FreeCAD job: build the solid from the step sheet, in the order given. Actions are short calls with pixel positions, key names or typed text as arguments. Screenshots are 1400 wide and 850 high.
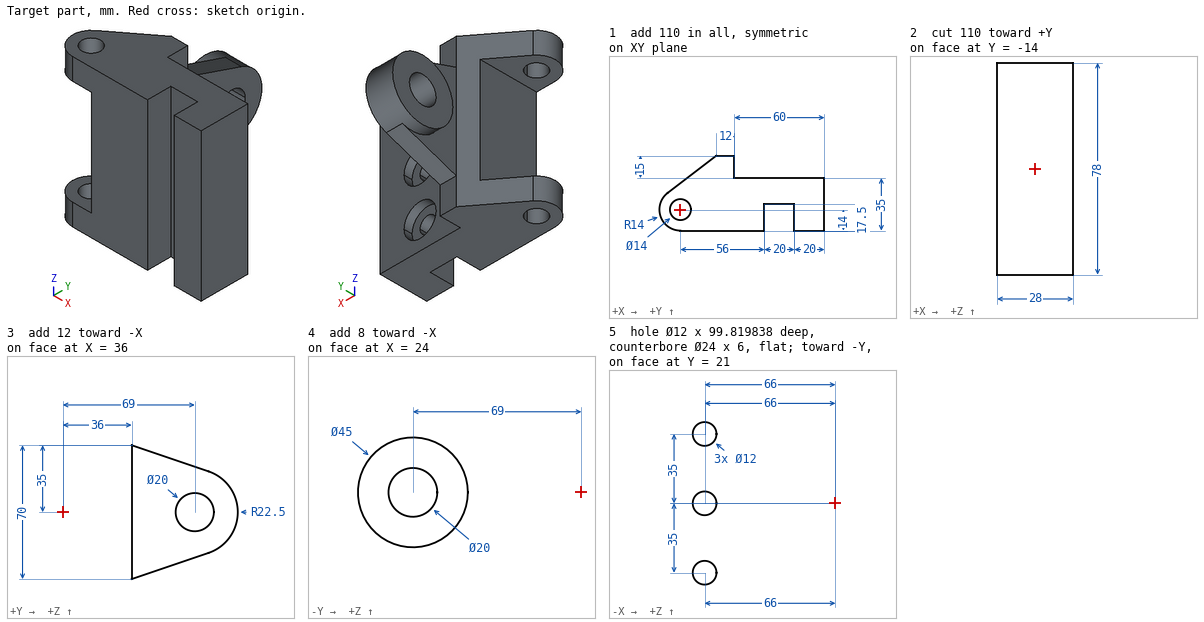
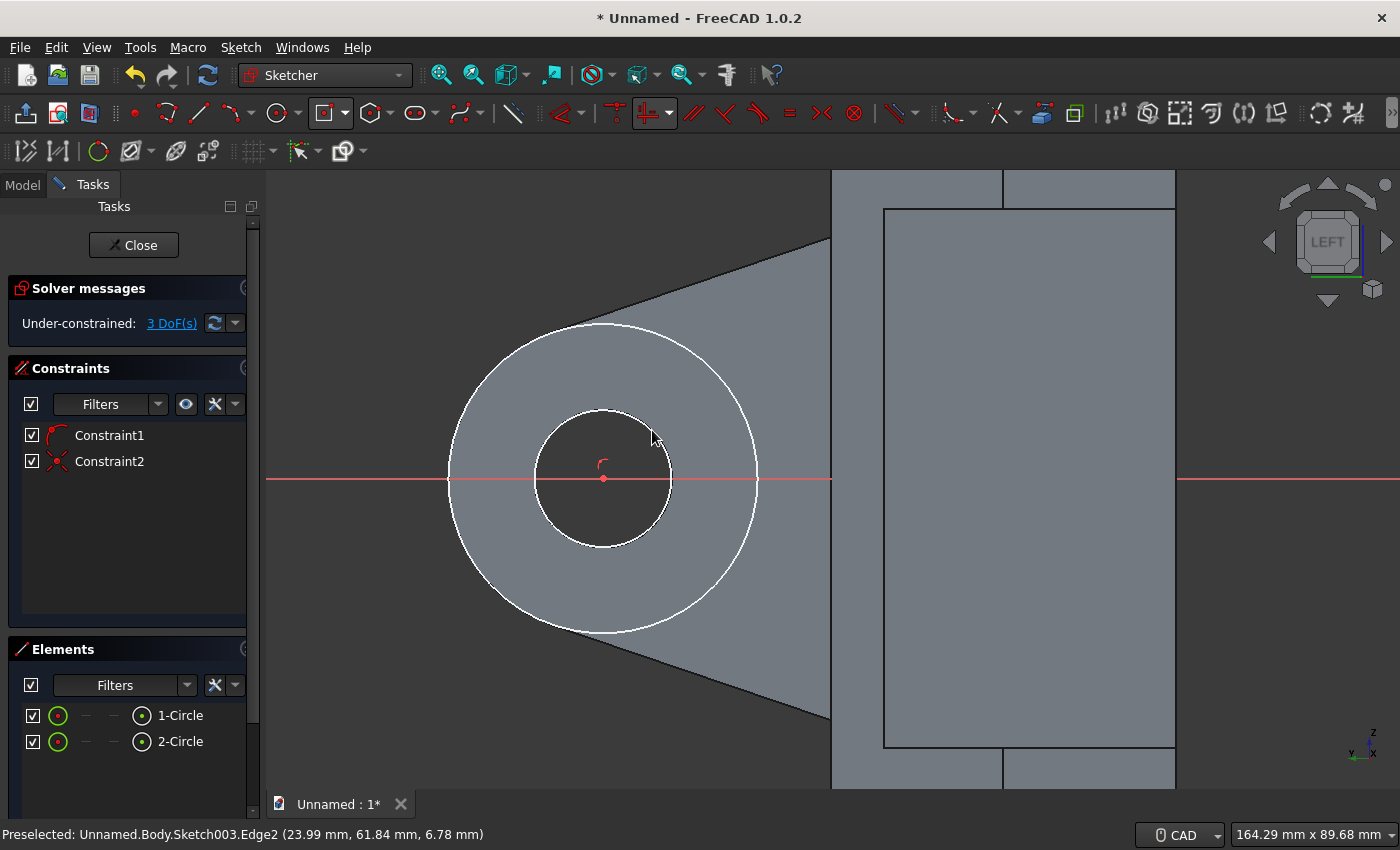
click(560, 114)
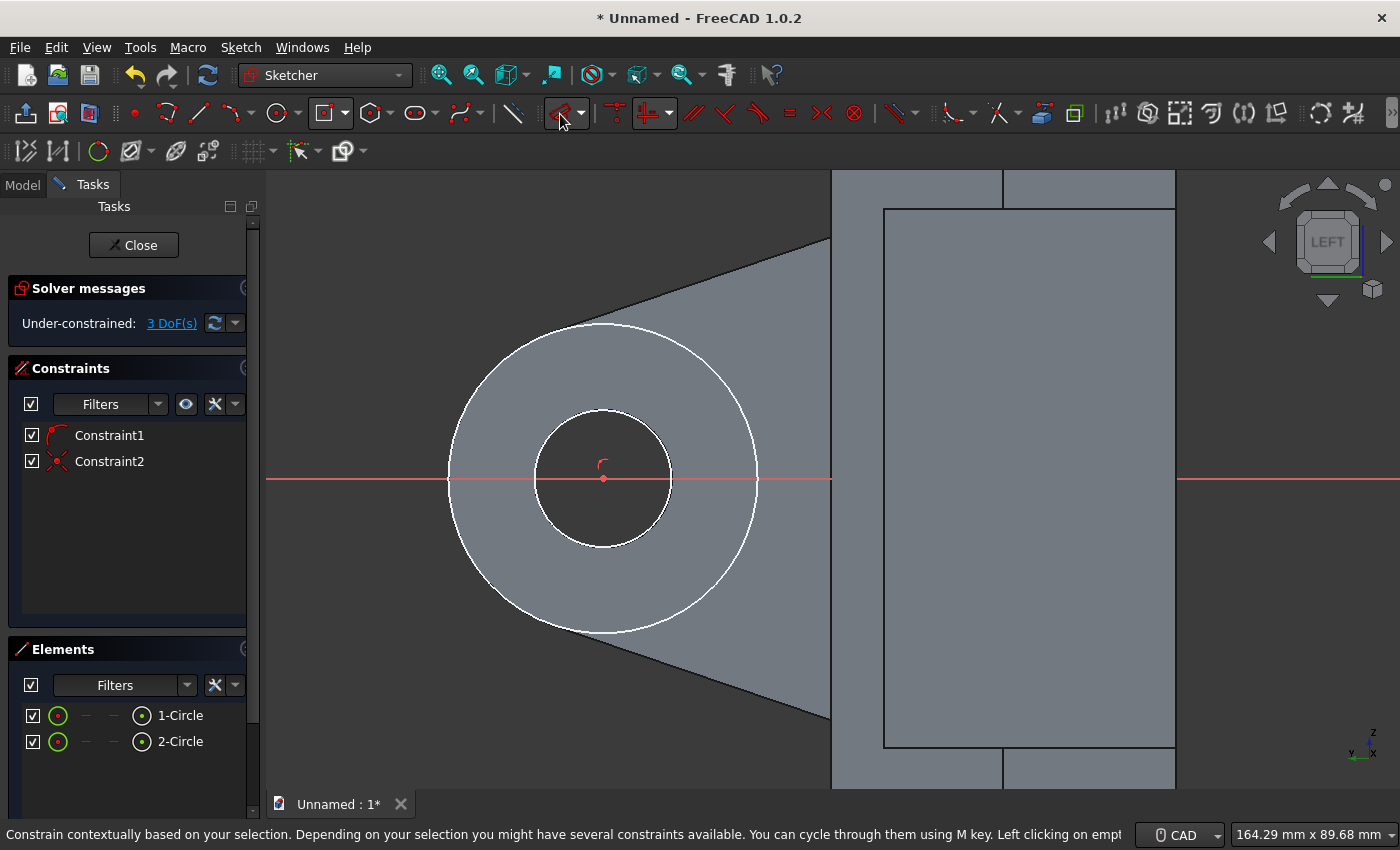
click(712, 369)
click(735, 346)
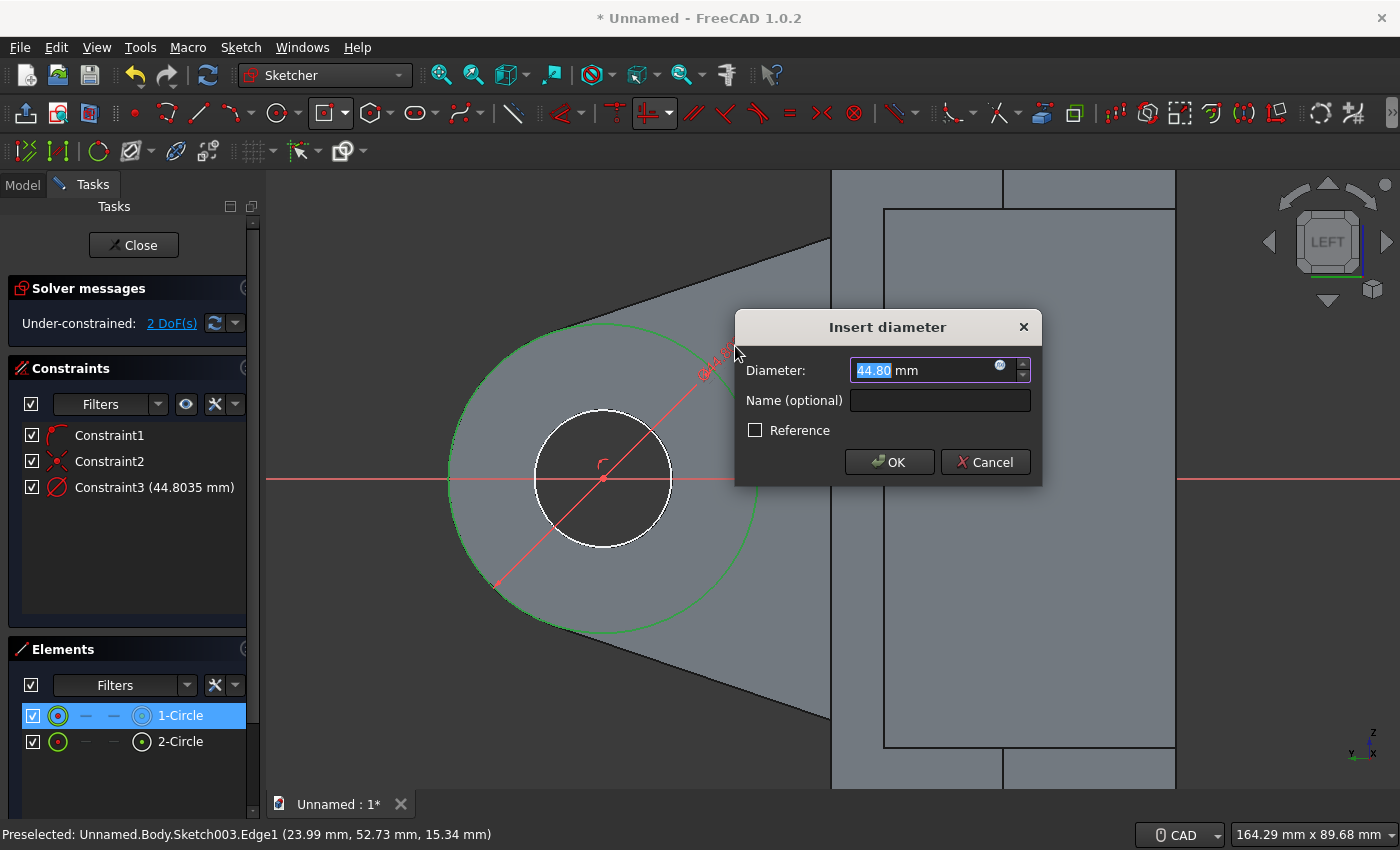
text(45)
key(Return)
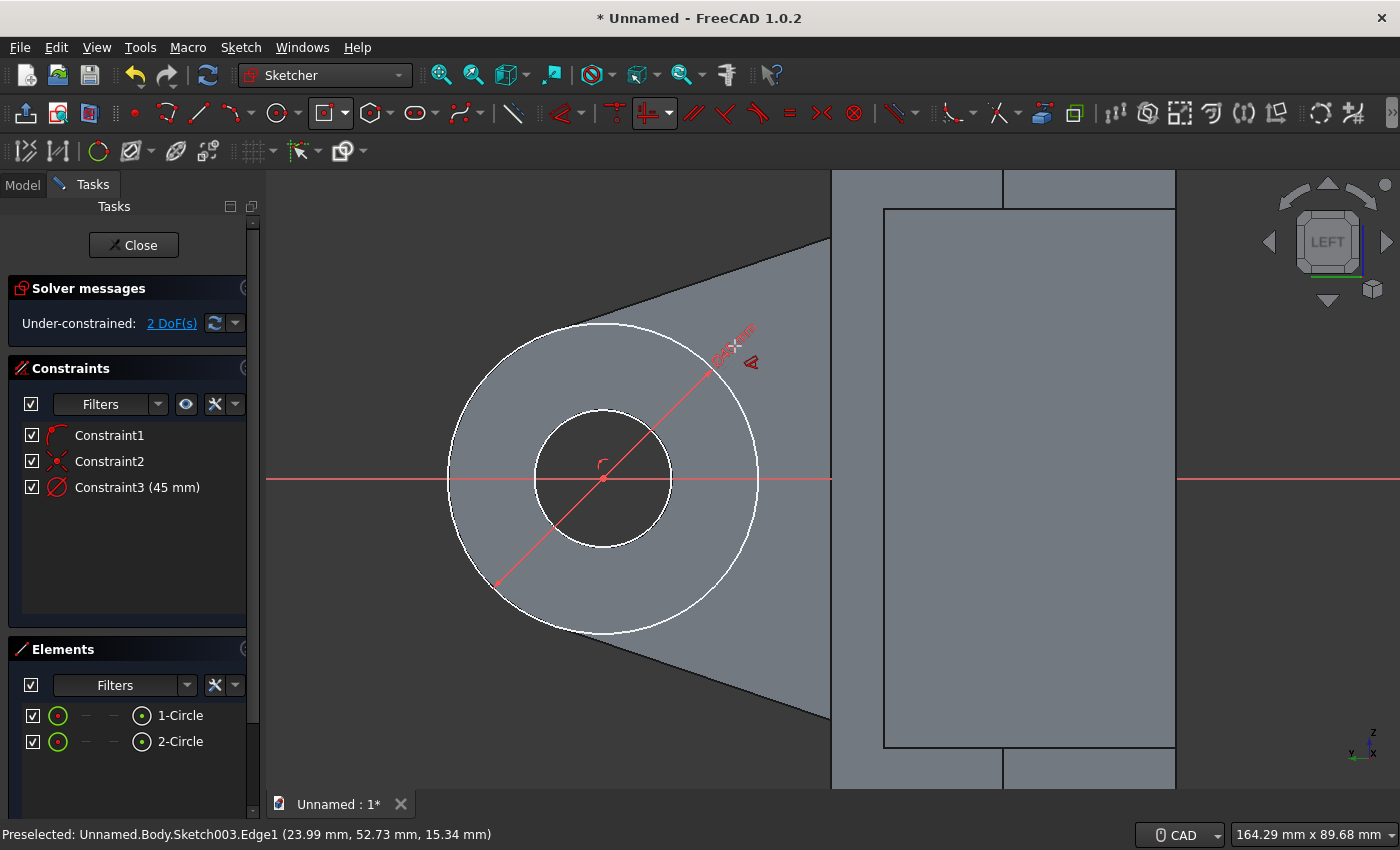
click(651, 430)
click(673, 407)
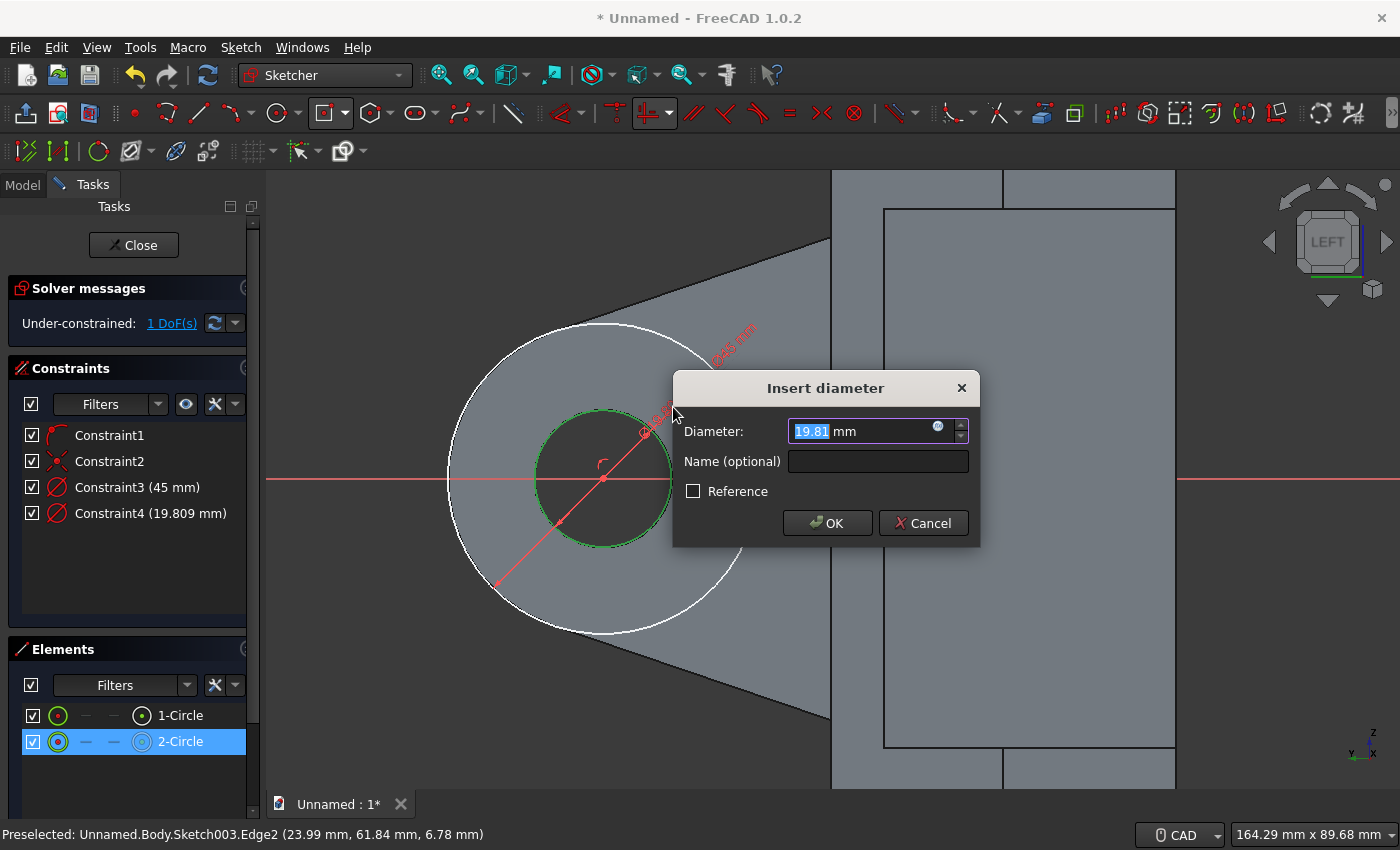
text(20)
key(Return)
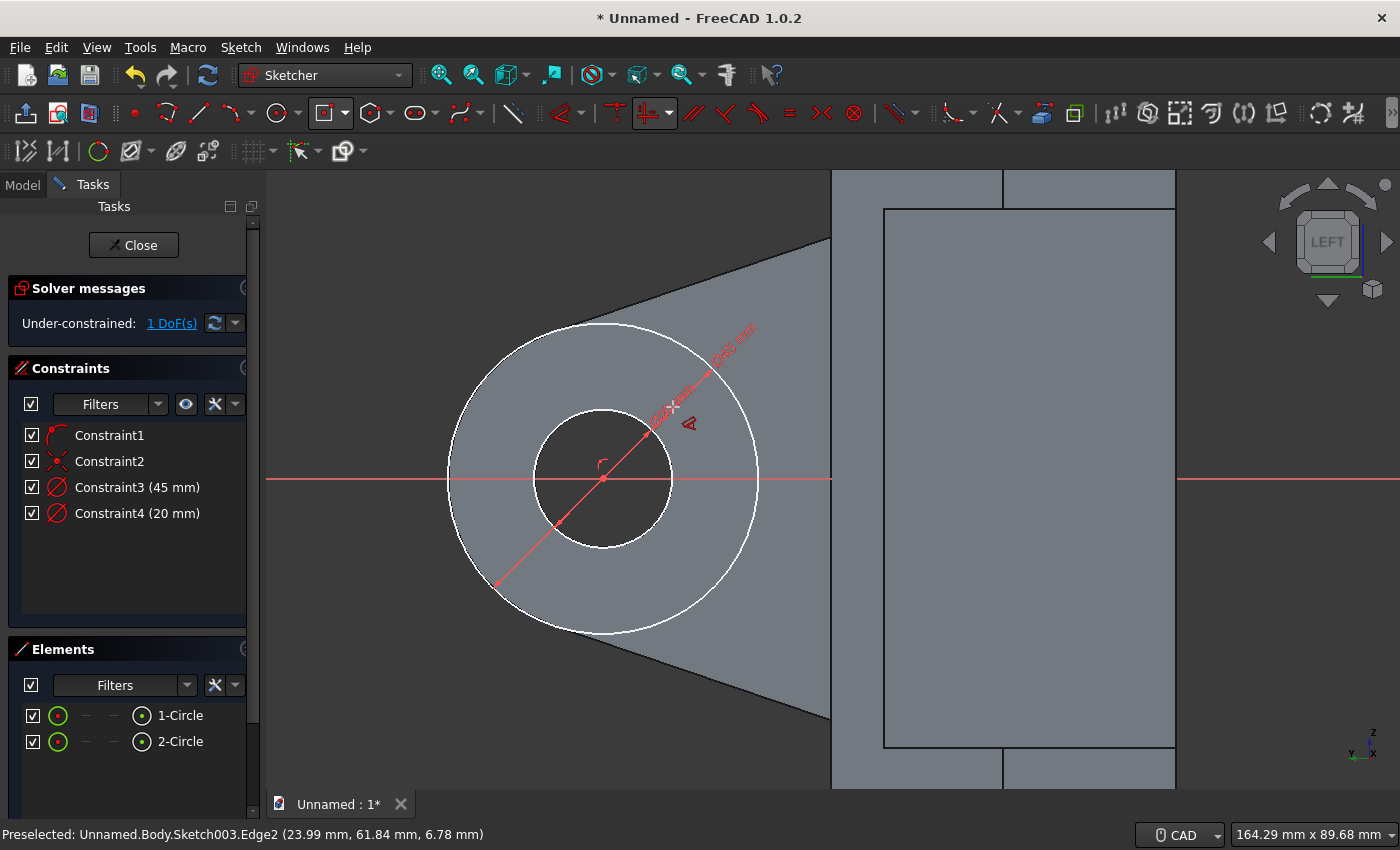
click(603, 479)
click(841, 513)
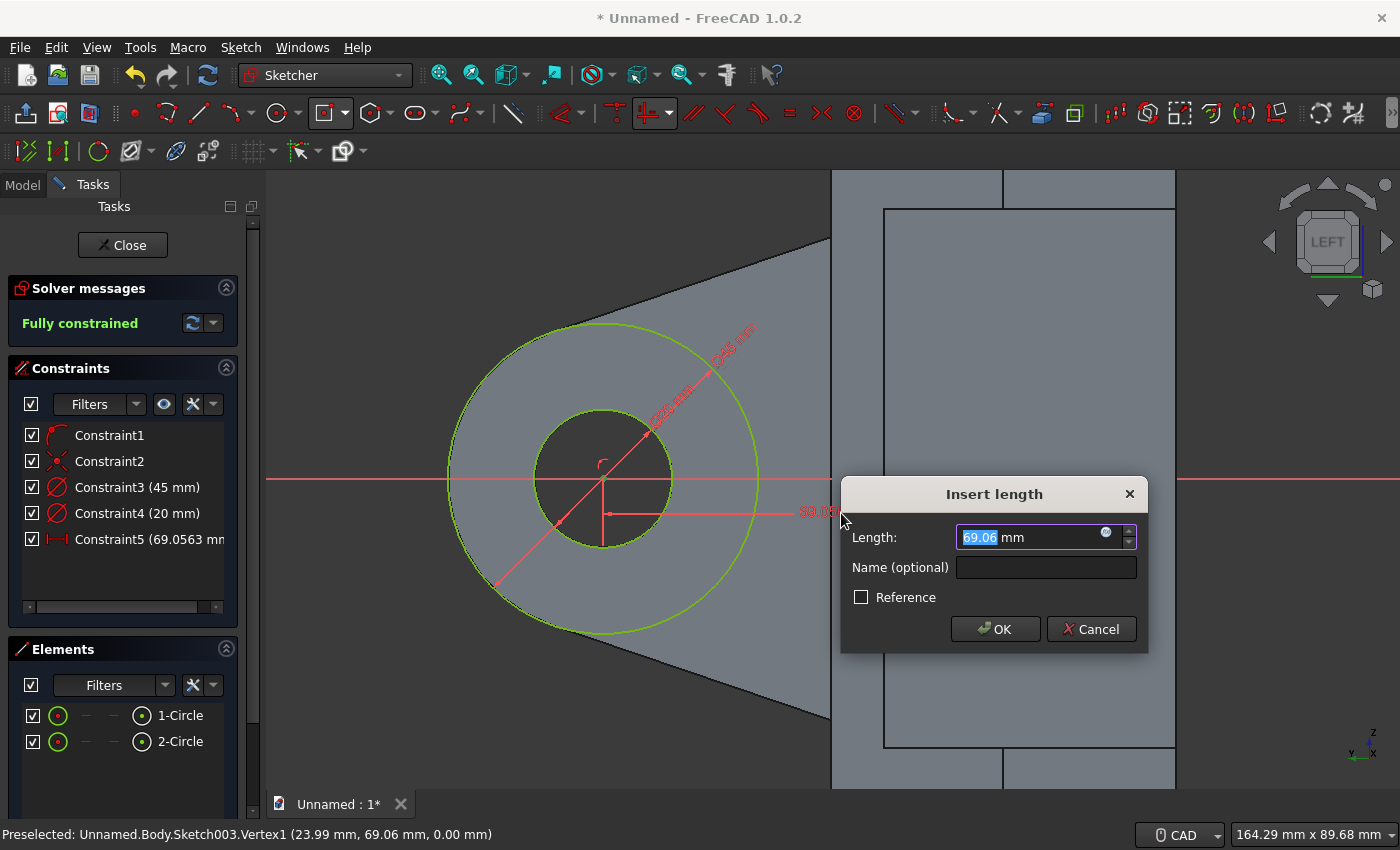
text(69)
key(Return)
key(Escape)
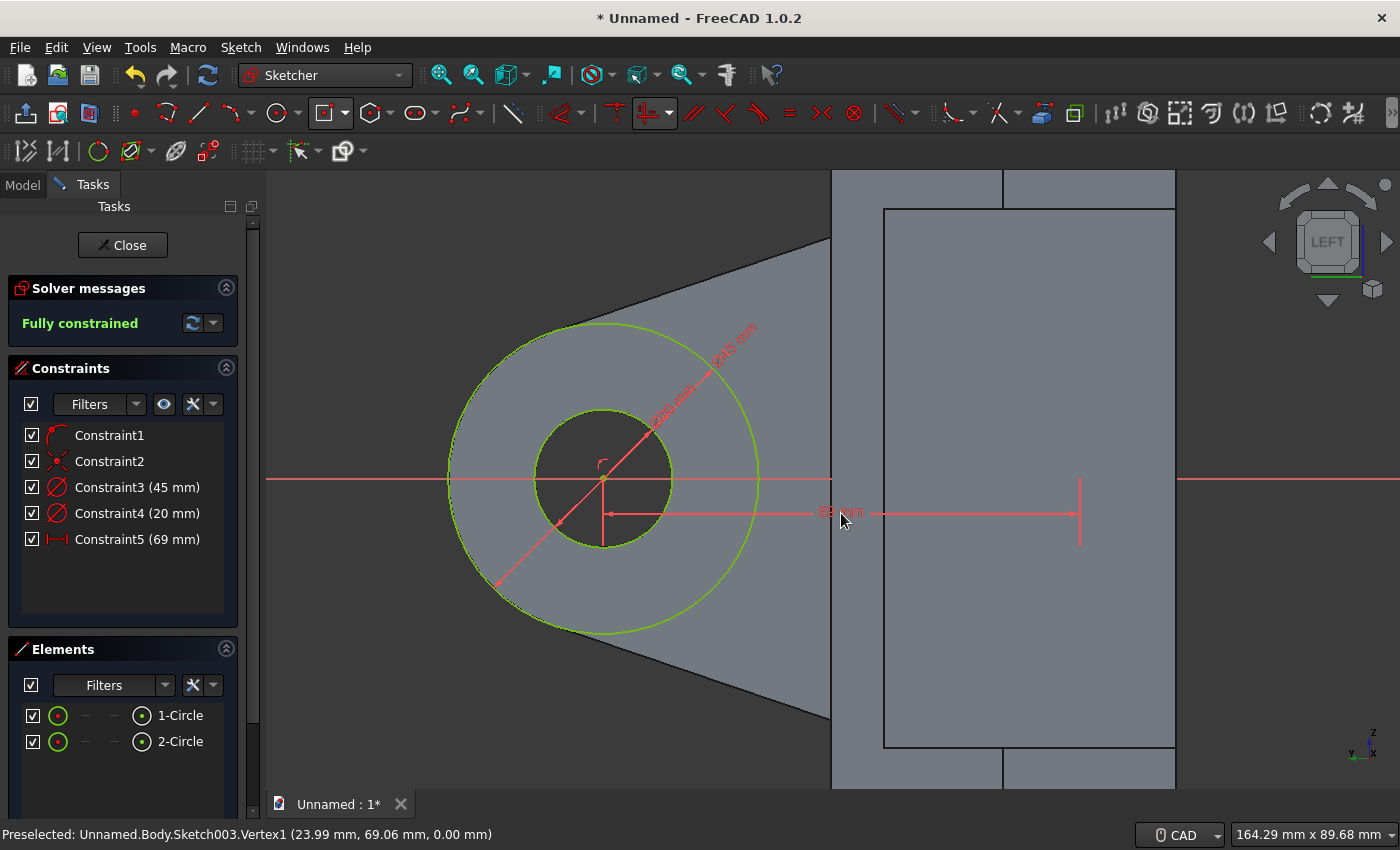
click(123, 245)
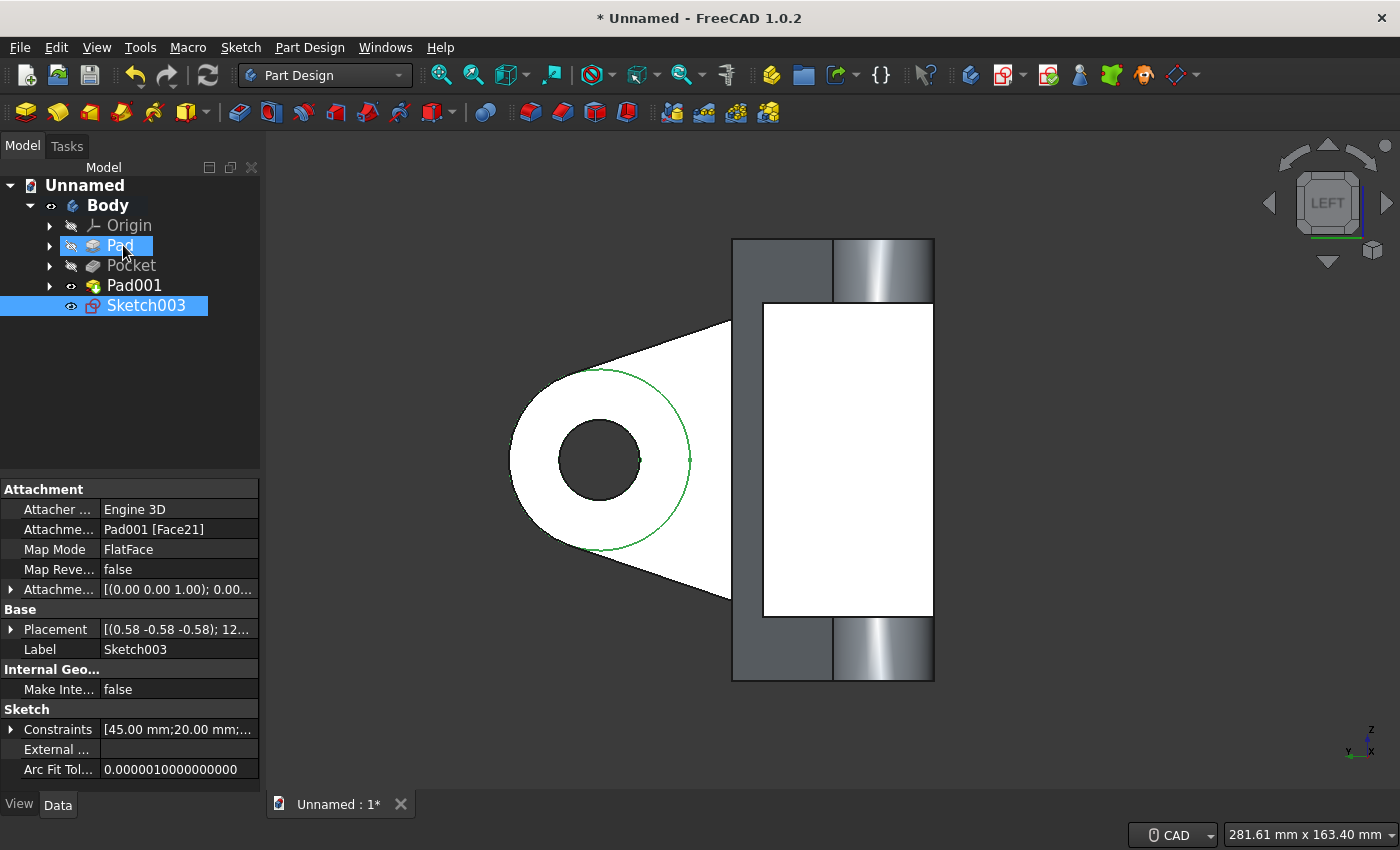
click(26, 112)